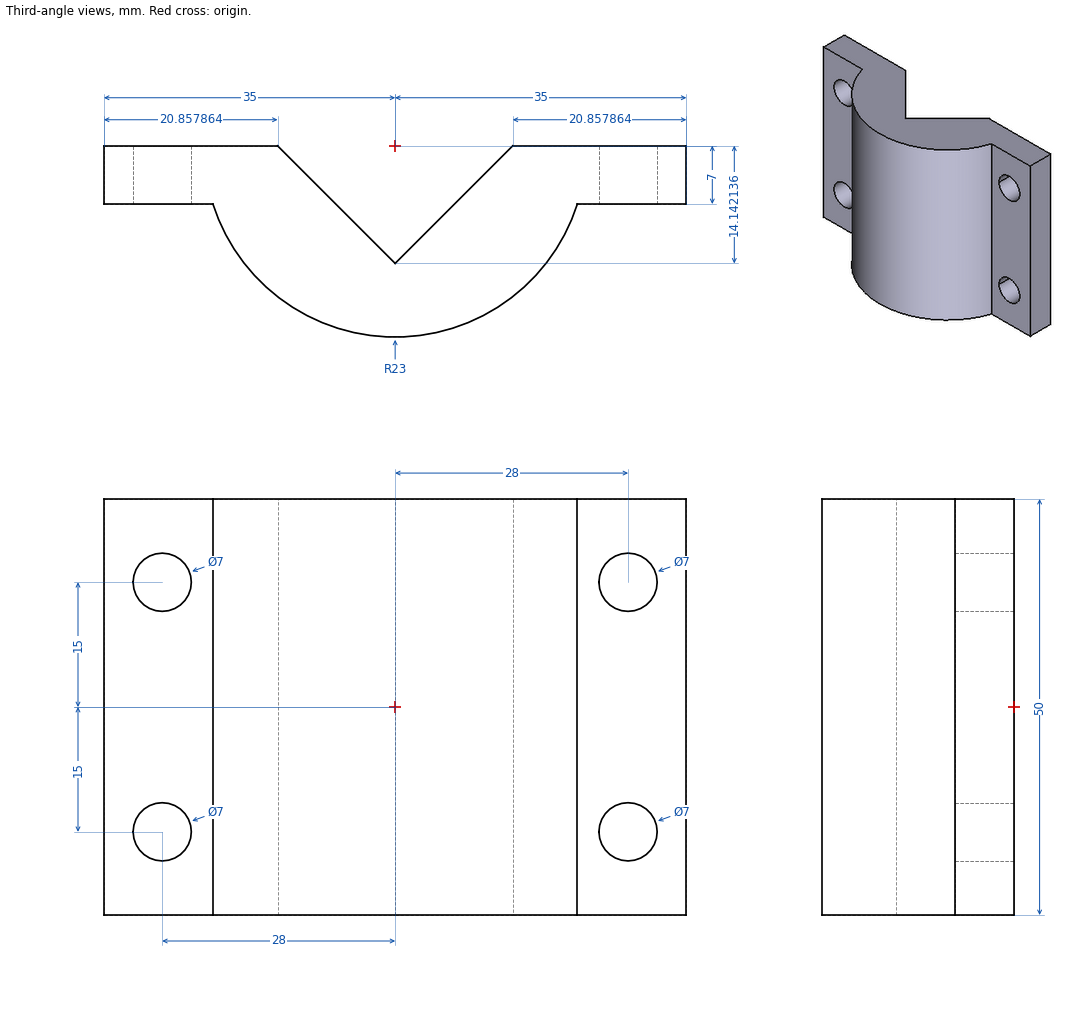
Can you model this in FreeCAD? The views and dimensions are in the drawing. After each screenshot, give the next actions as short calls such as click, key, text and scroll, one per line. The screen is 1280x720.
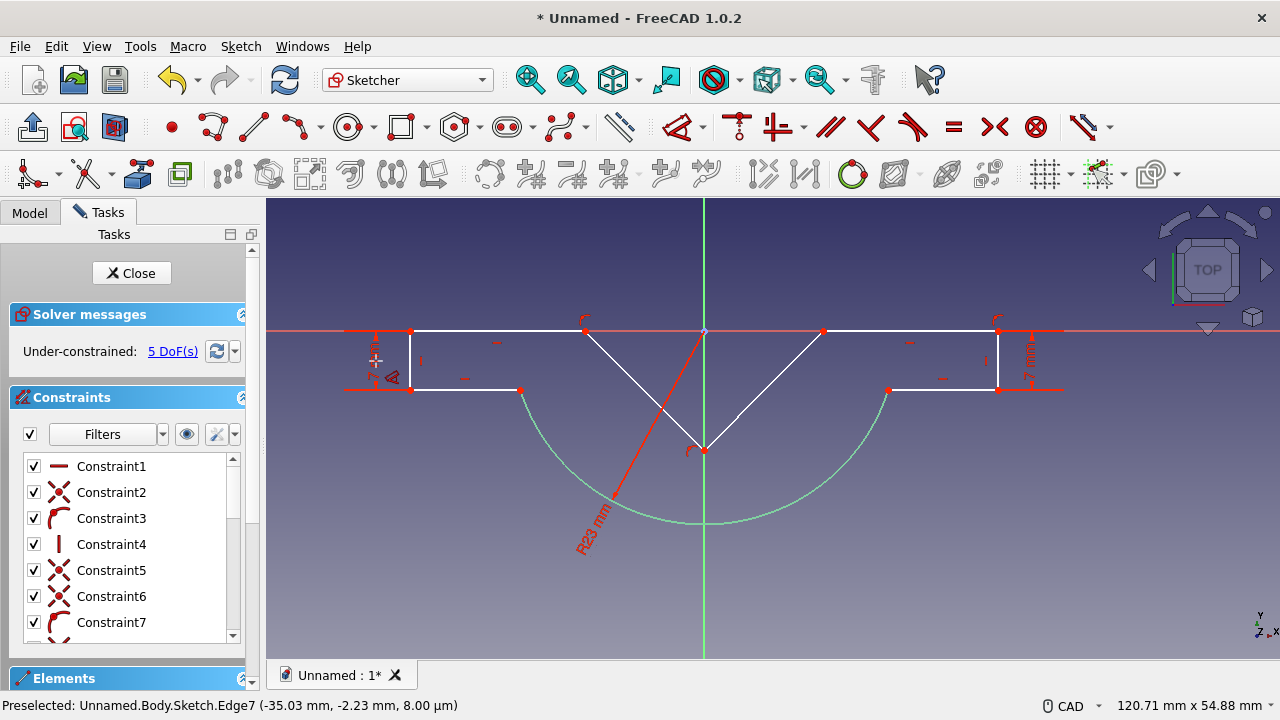
click(998, 390)
click(851, 297)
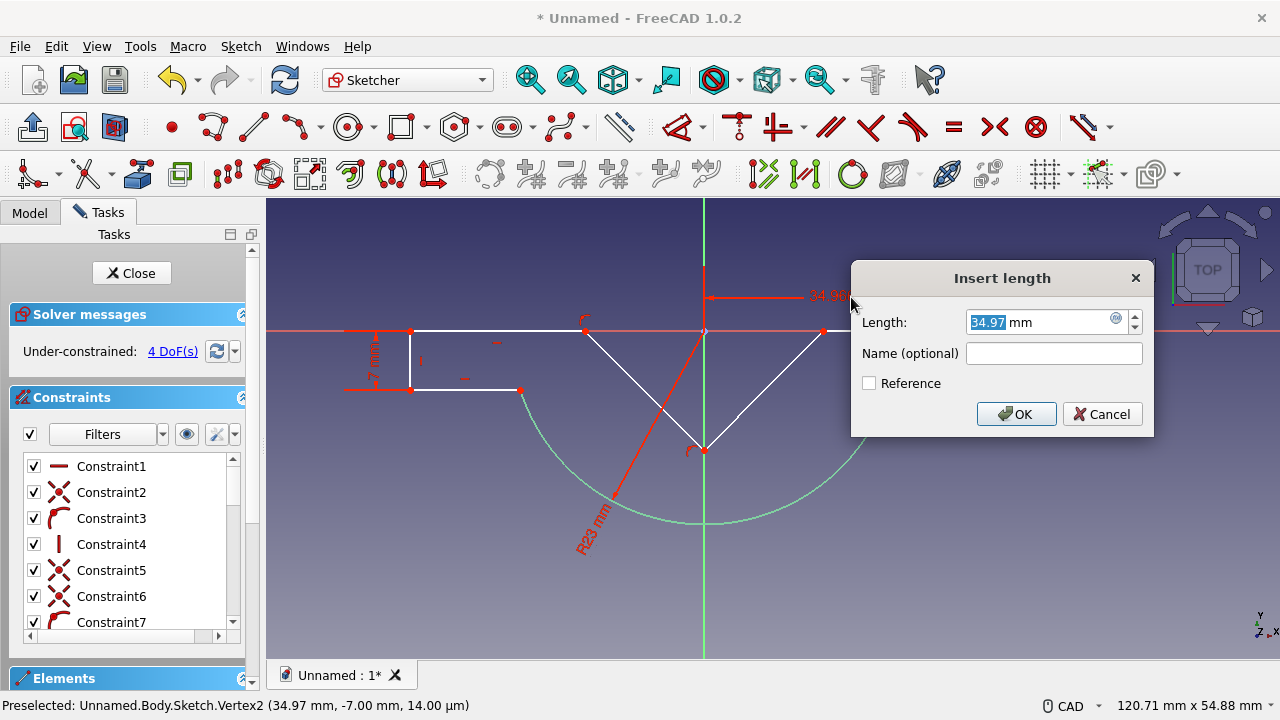
text(35)
key(Return)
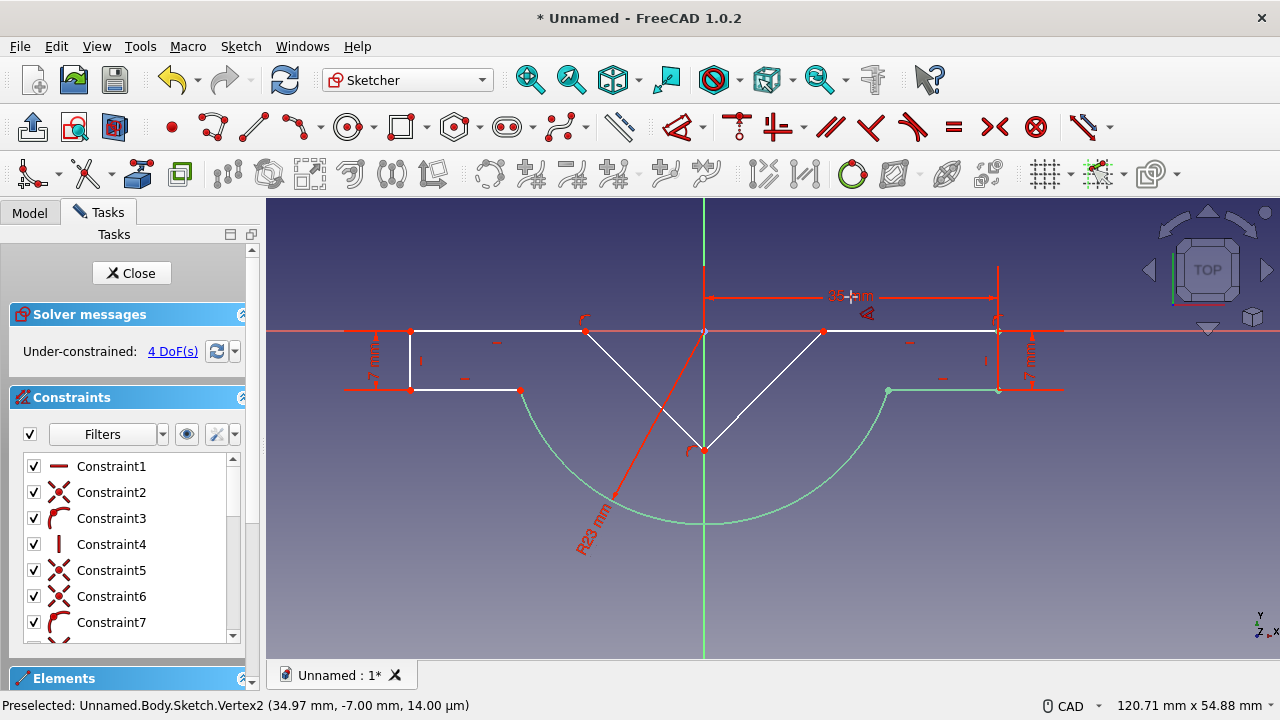
click(410, 331)
click(557, 297)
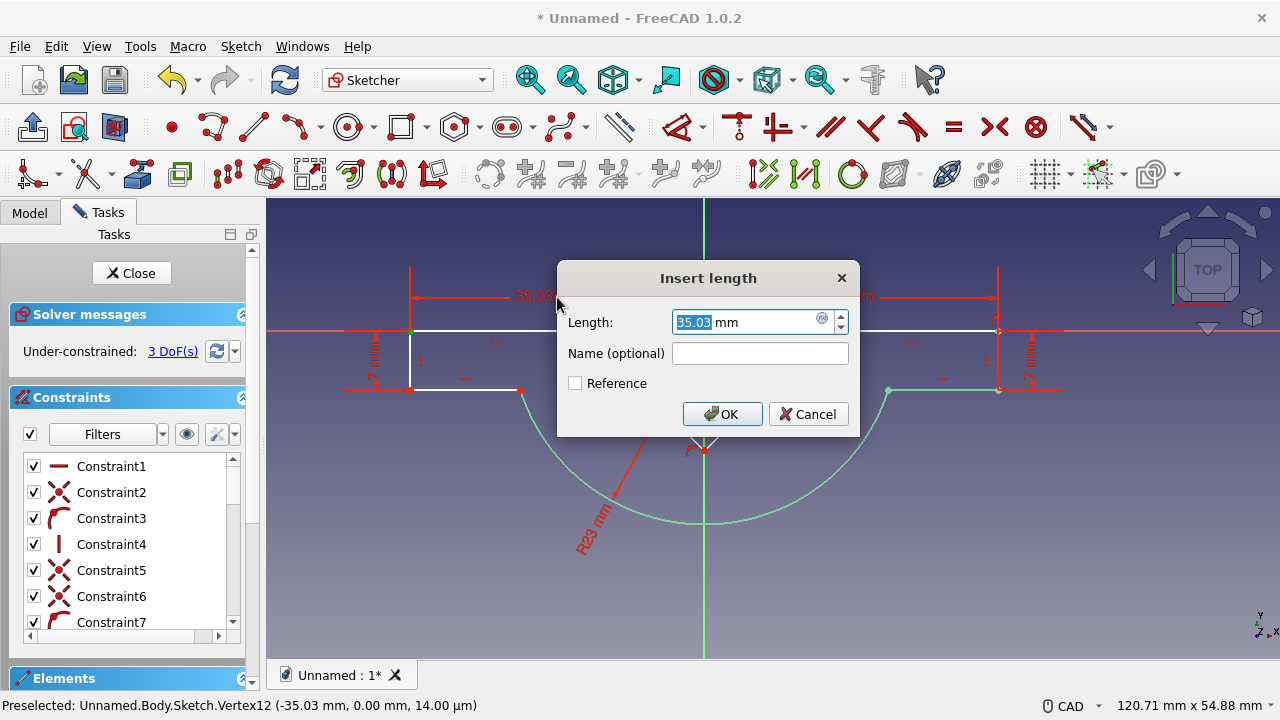
text(35)
key(Return)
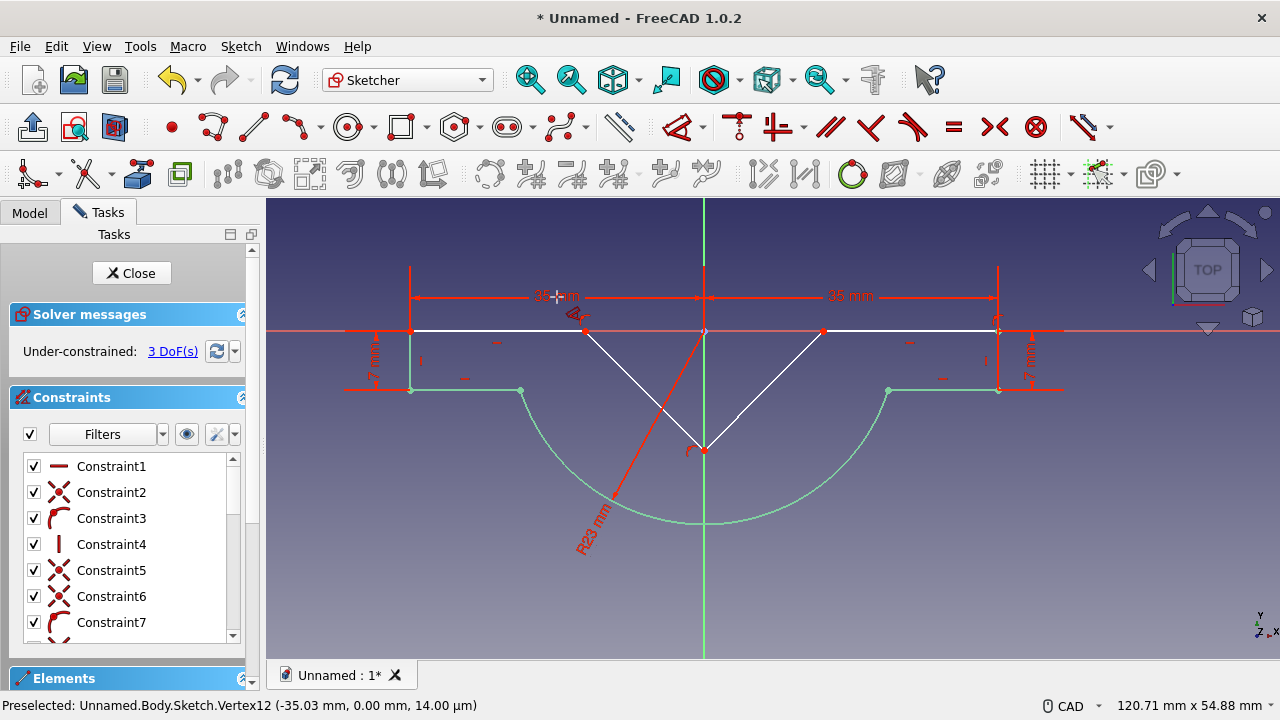
click(946, 331)
click(951, 297)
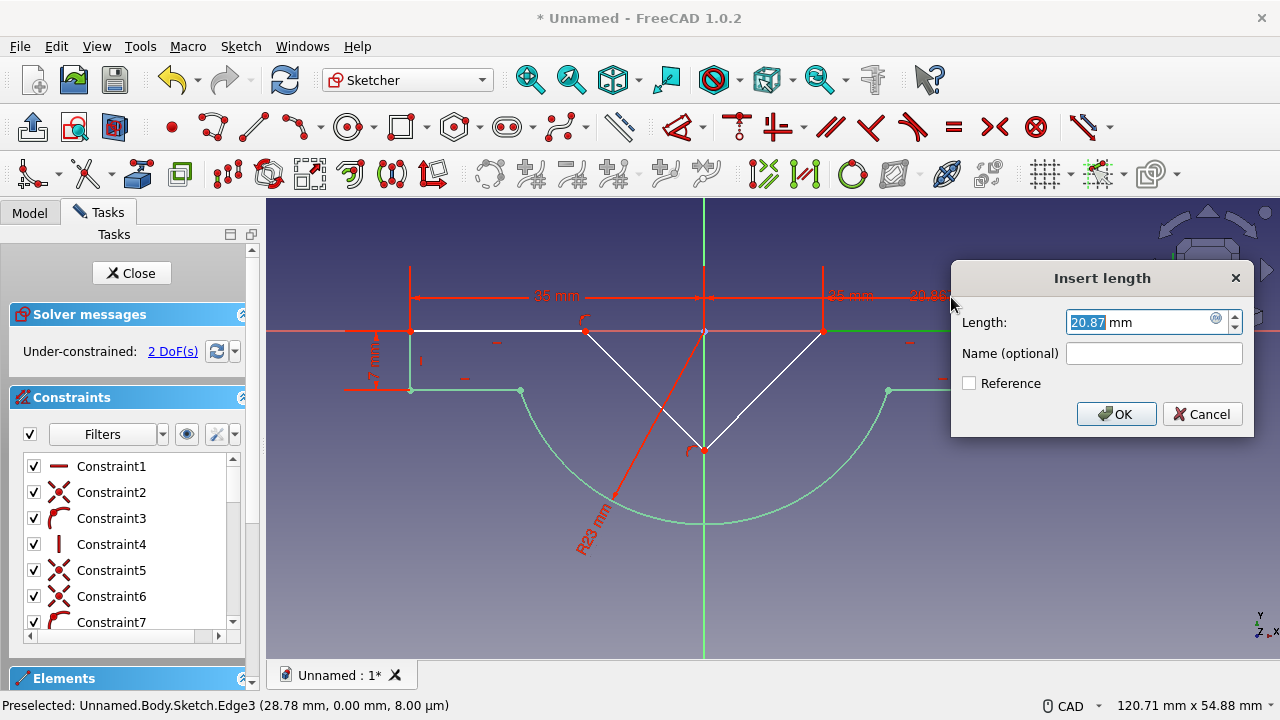
text(20.857864)
key(Return)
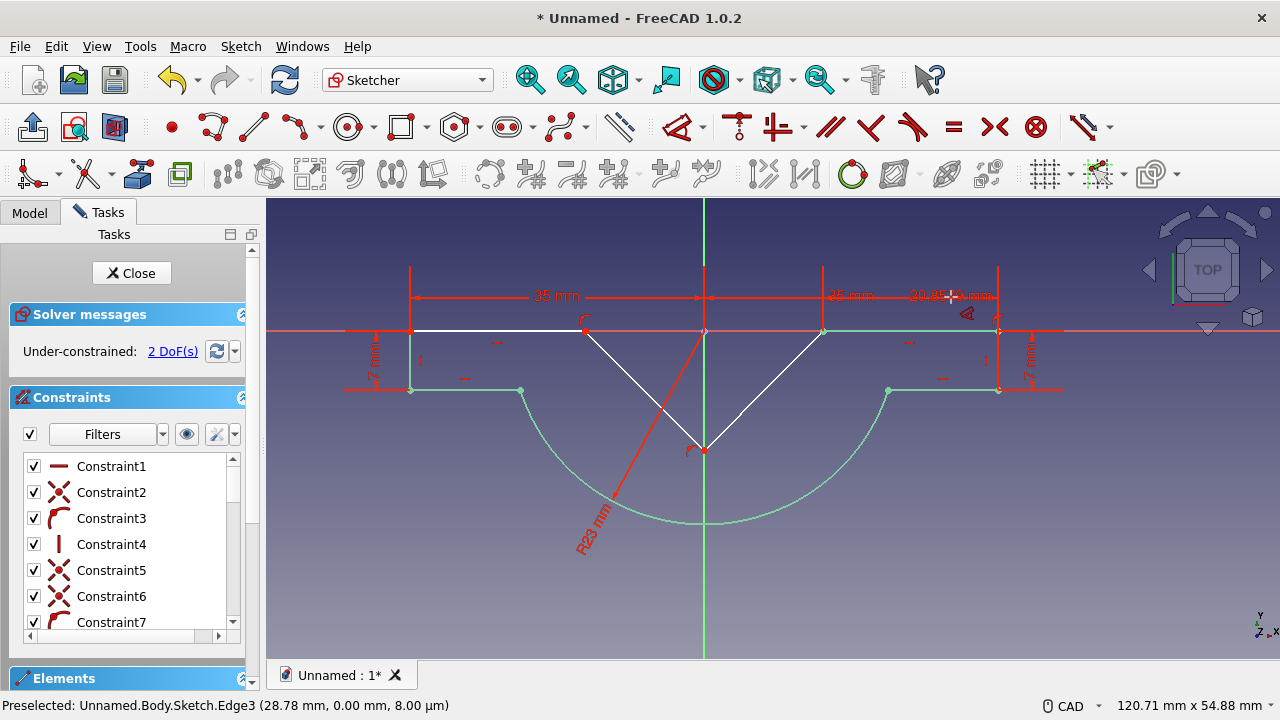
click(533, 331)
click(457, 297)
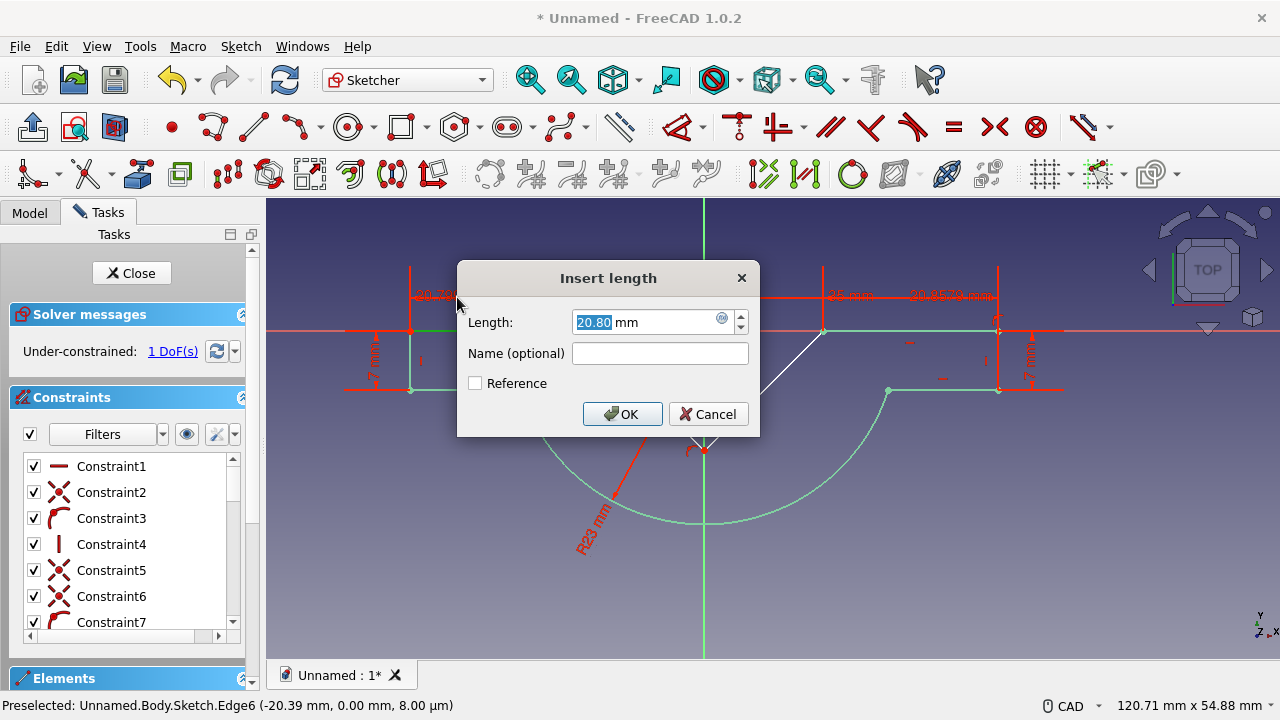
text(20.857864)
key(Return)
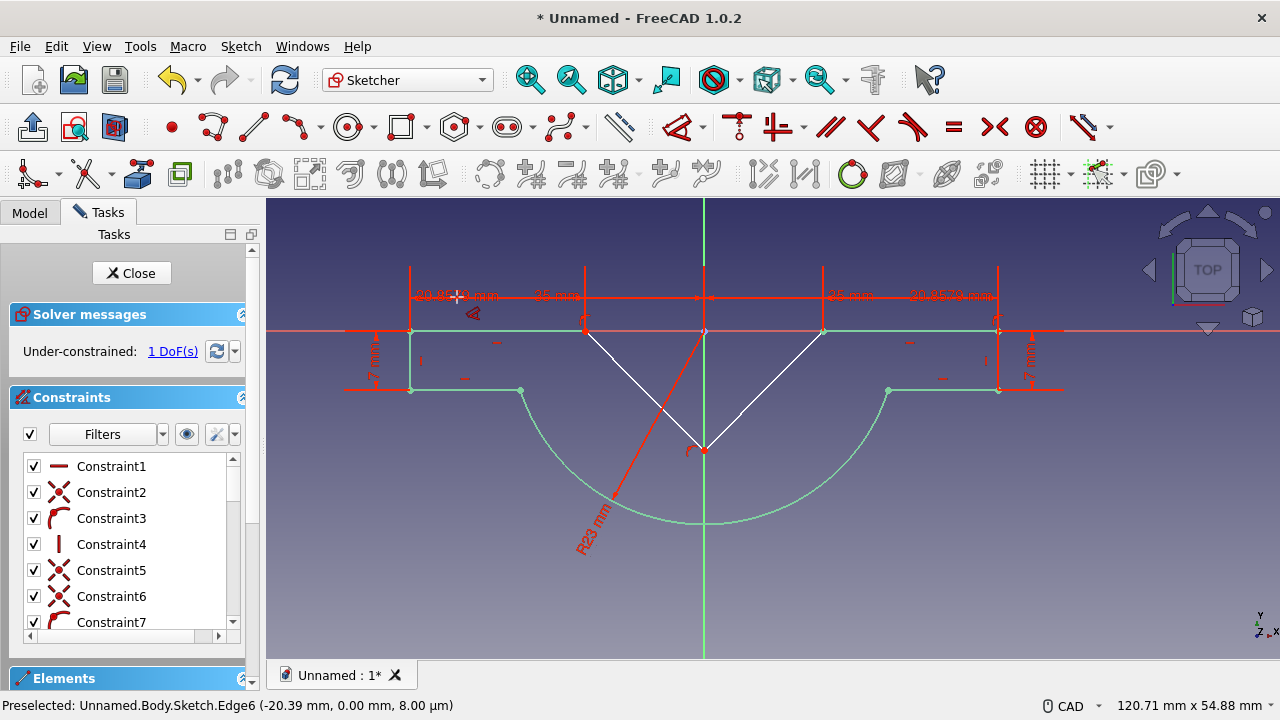
click(704, 451)
click(738, 391)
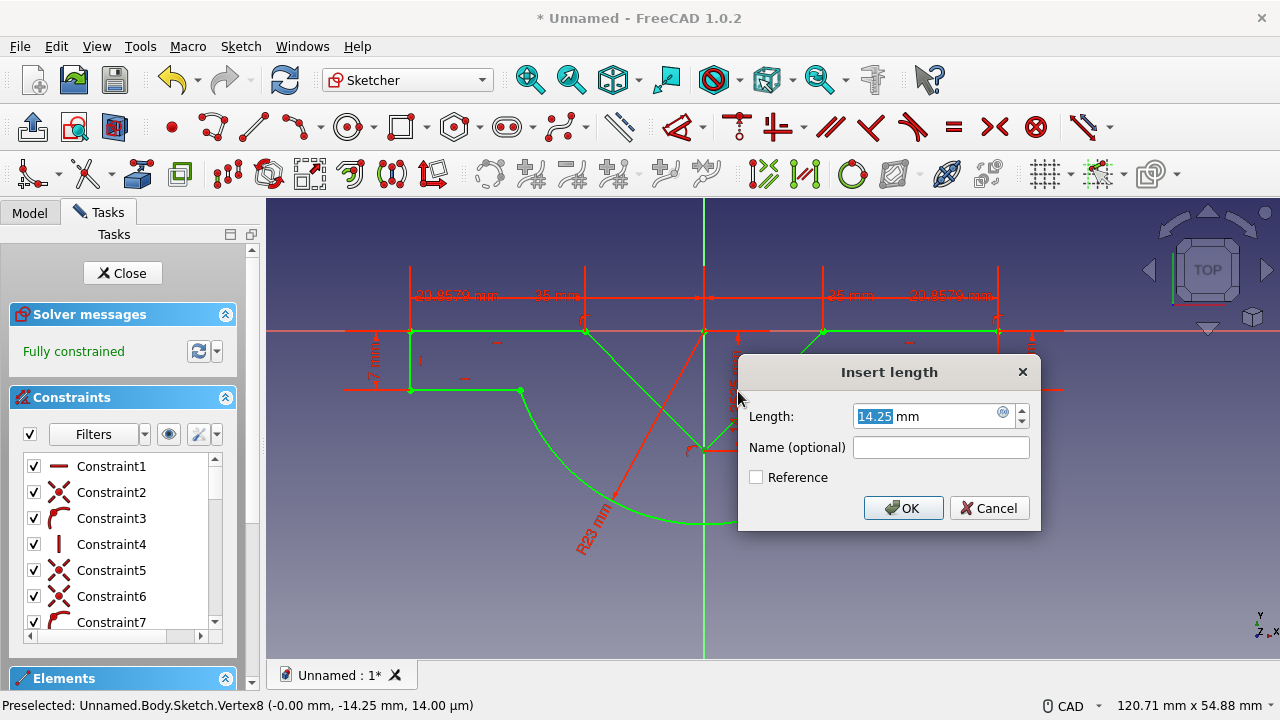
text(14.142136)
key(Return)
key(Escape)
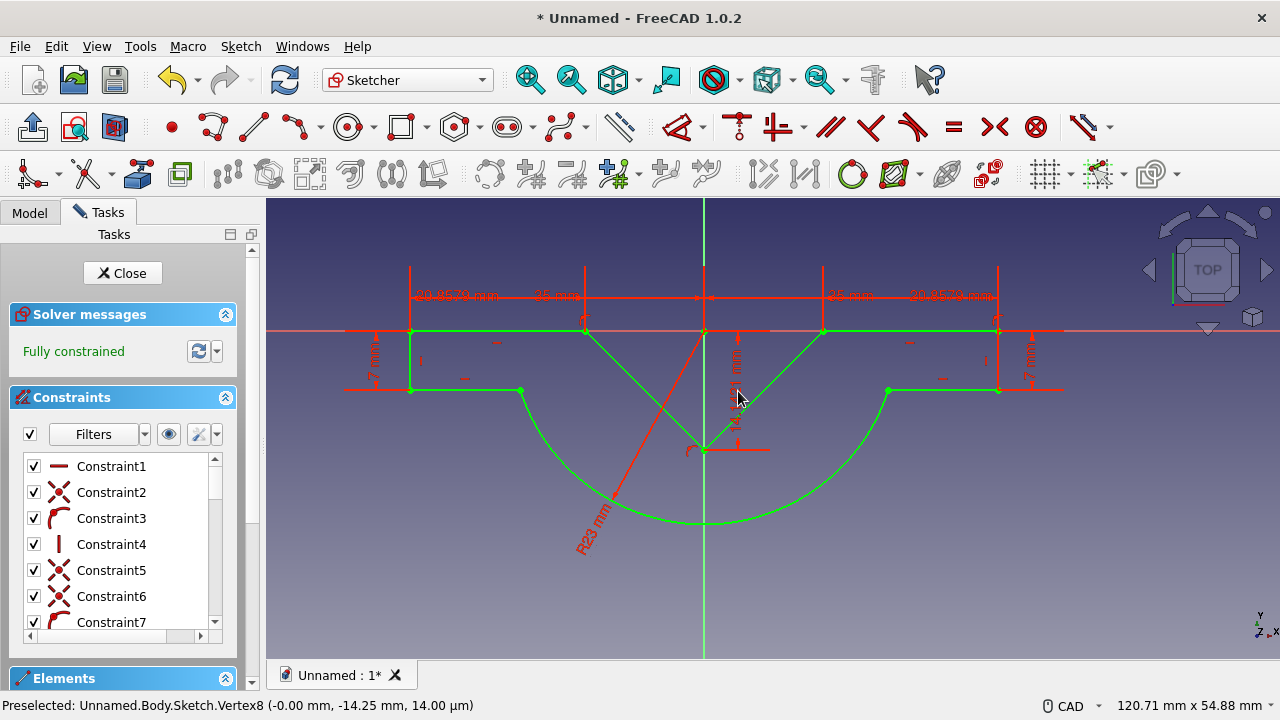
click(123, 273)